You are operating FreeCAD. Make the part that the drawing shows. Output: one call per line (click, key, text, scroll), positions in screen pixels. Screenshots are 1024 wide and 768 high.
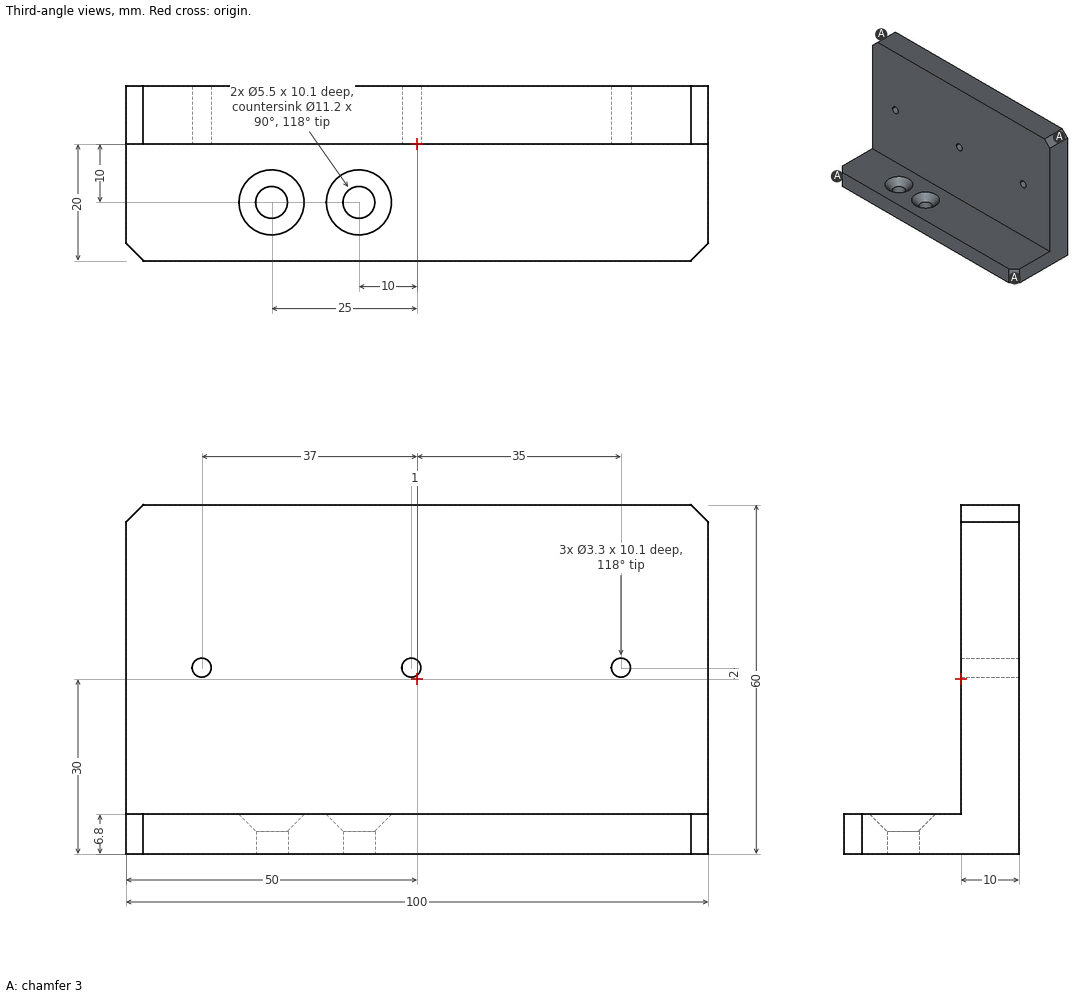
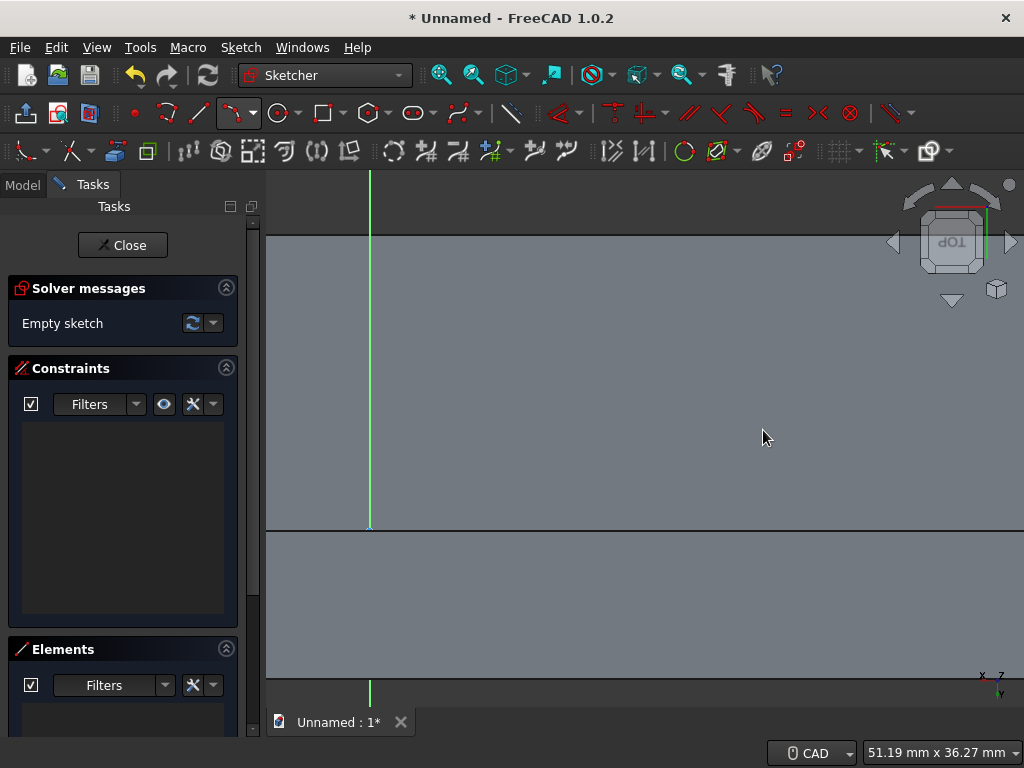
key(g)
key(c)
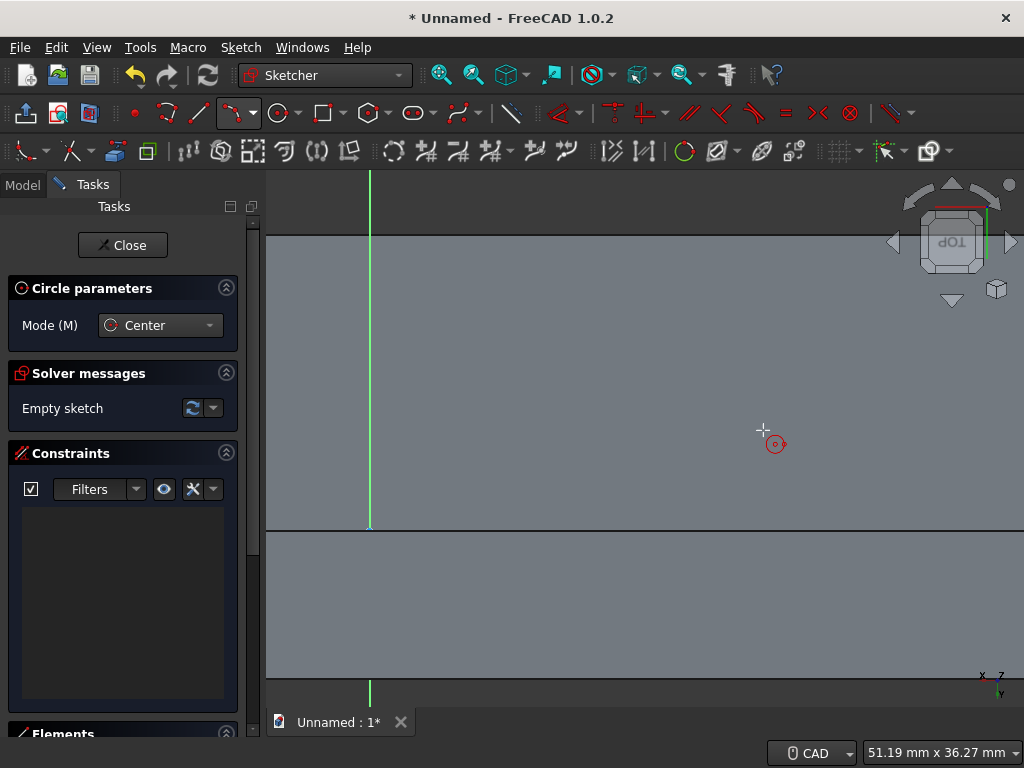
click(518, 383)
click(547, 354)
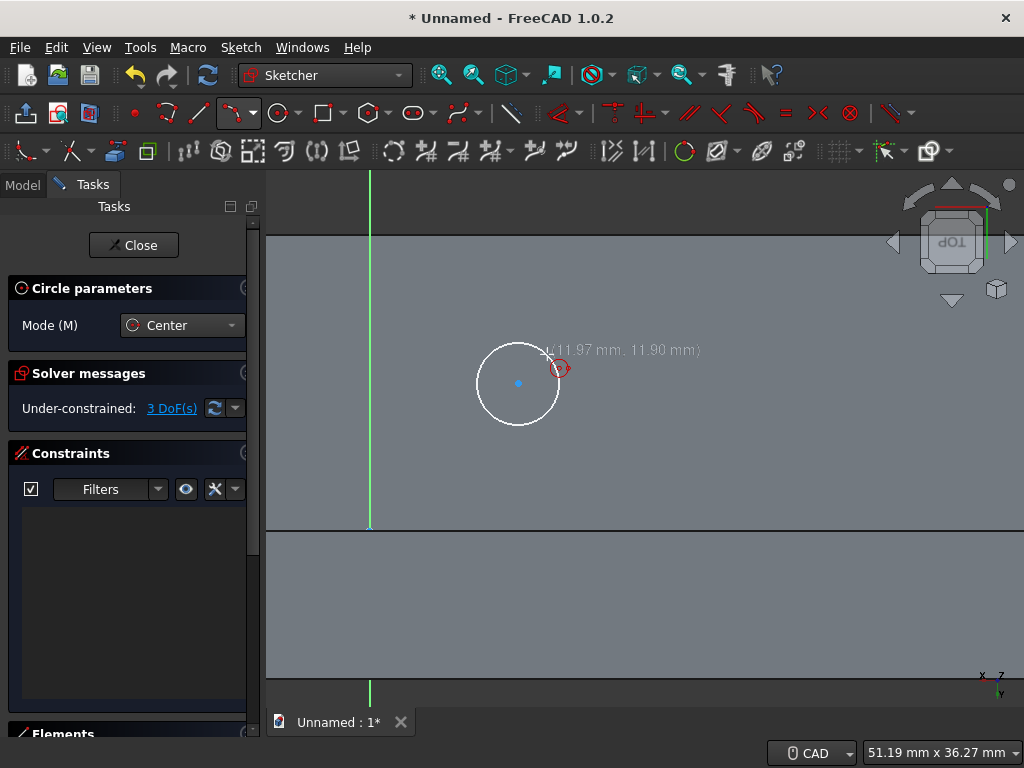
click(740, 383)
click(769, 354)
key(Escape)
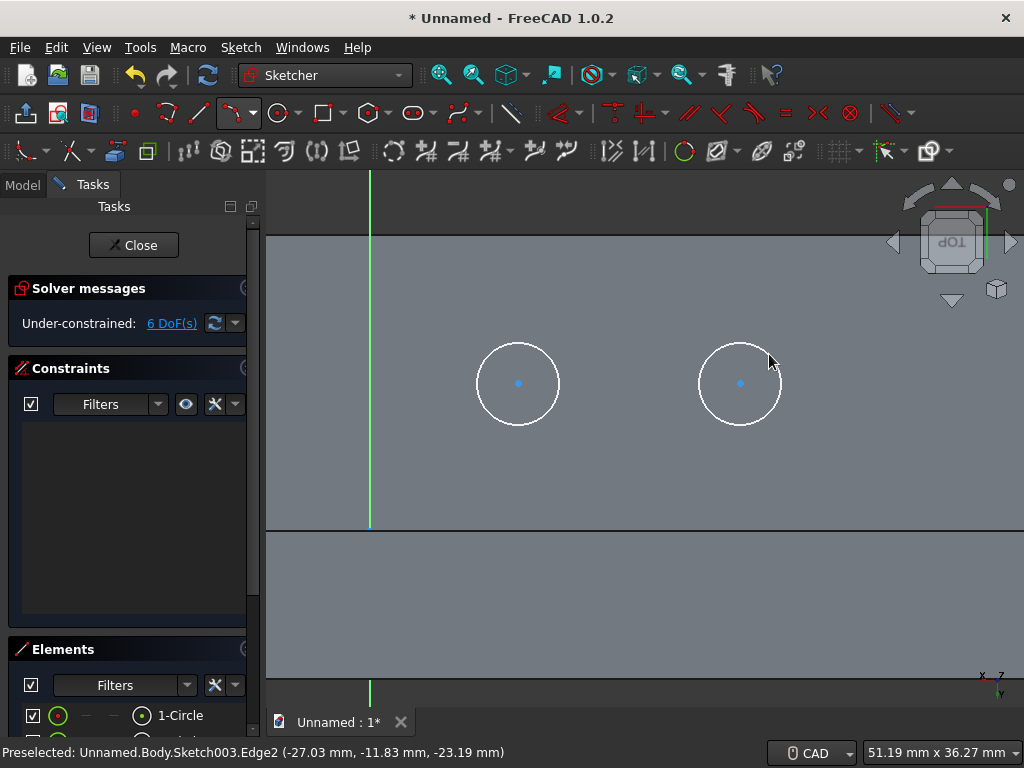
click(547, 355)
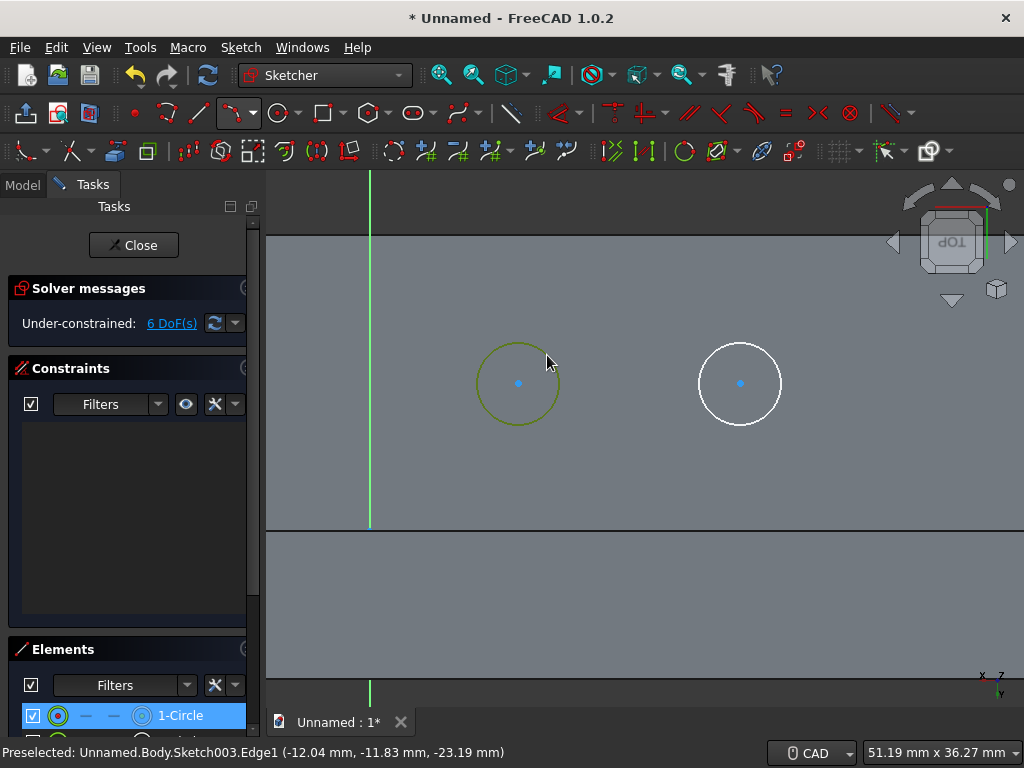
click(769, 355)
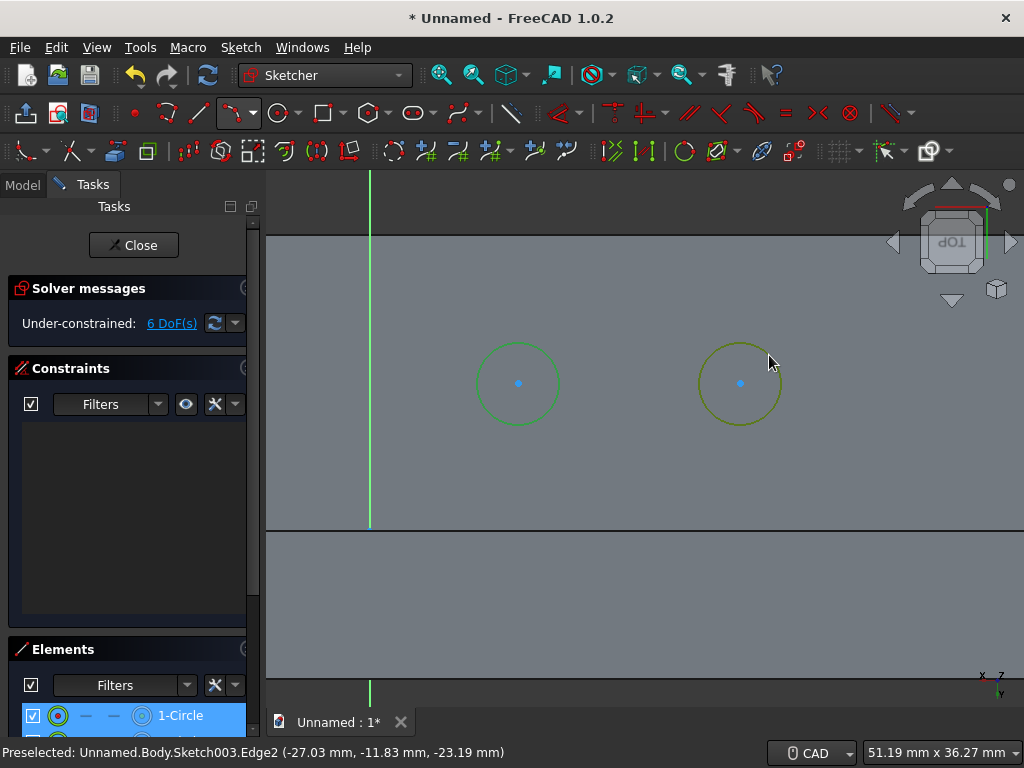
click(786, 114)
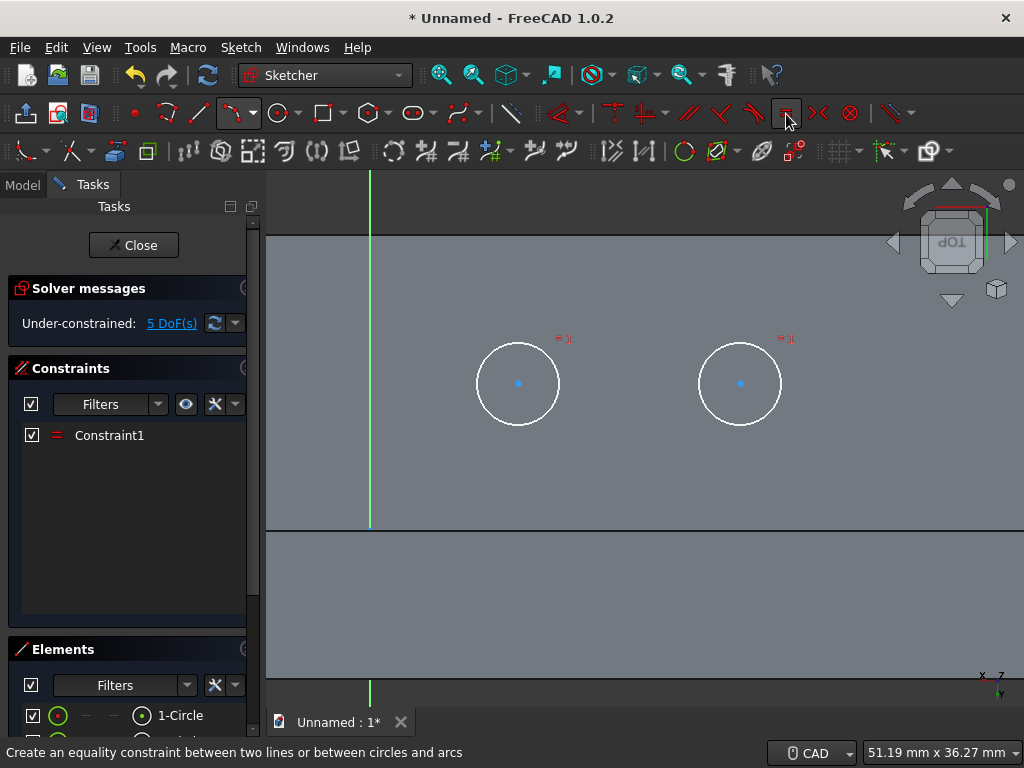
click(518, 384)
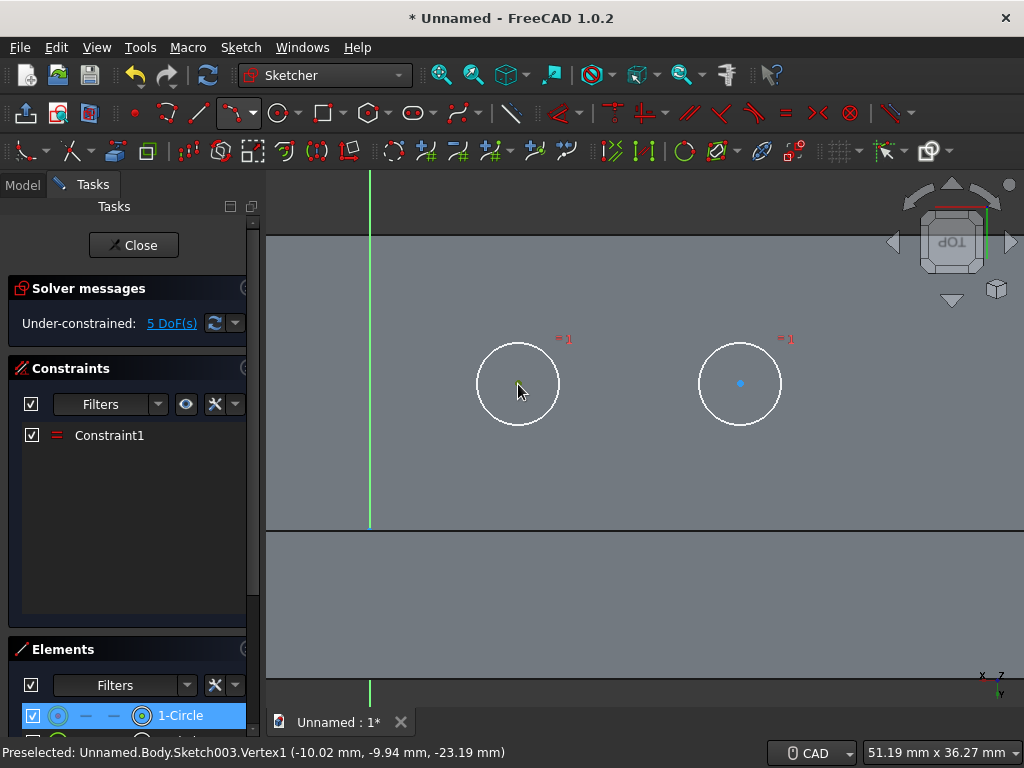
click(740, 384)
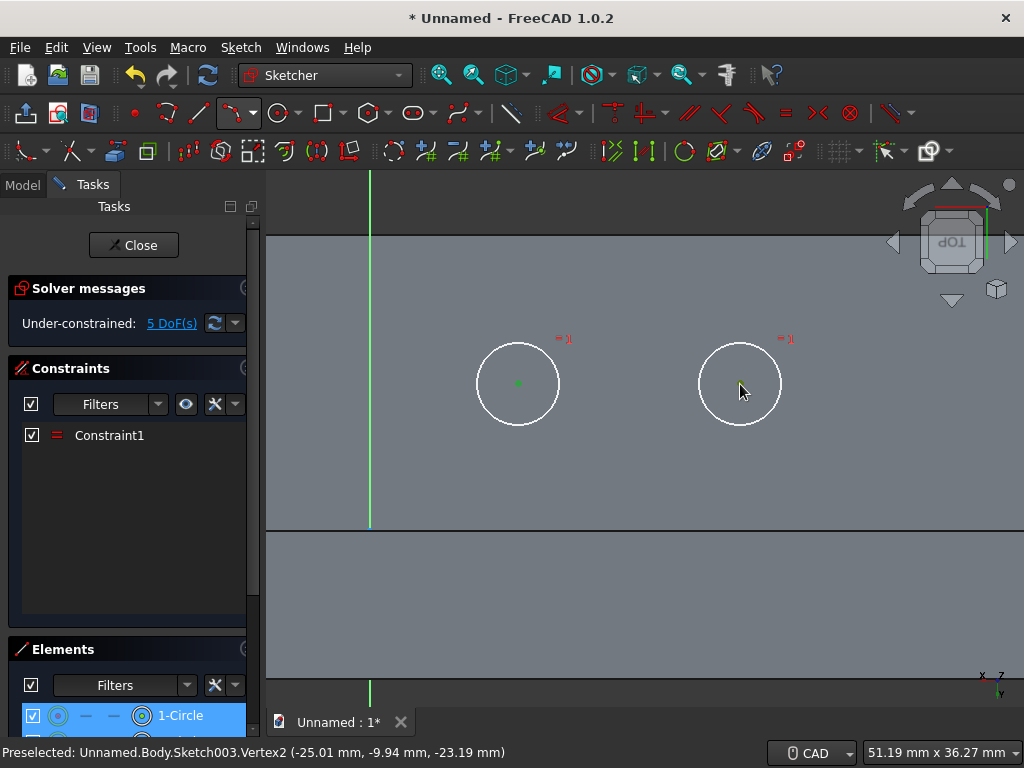
key(h)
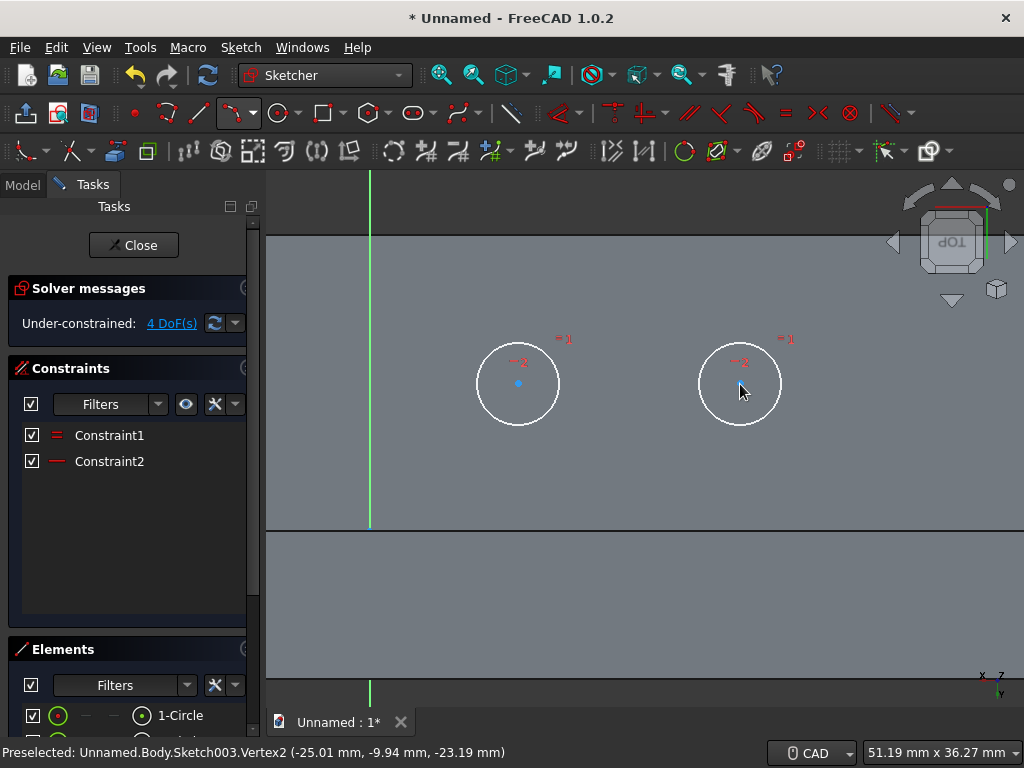
key(d)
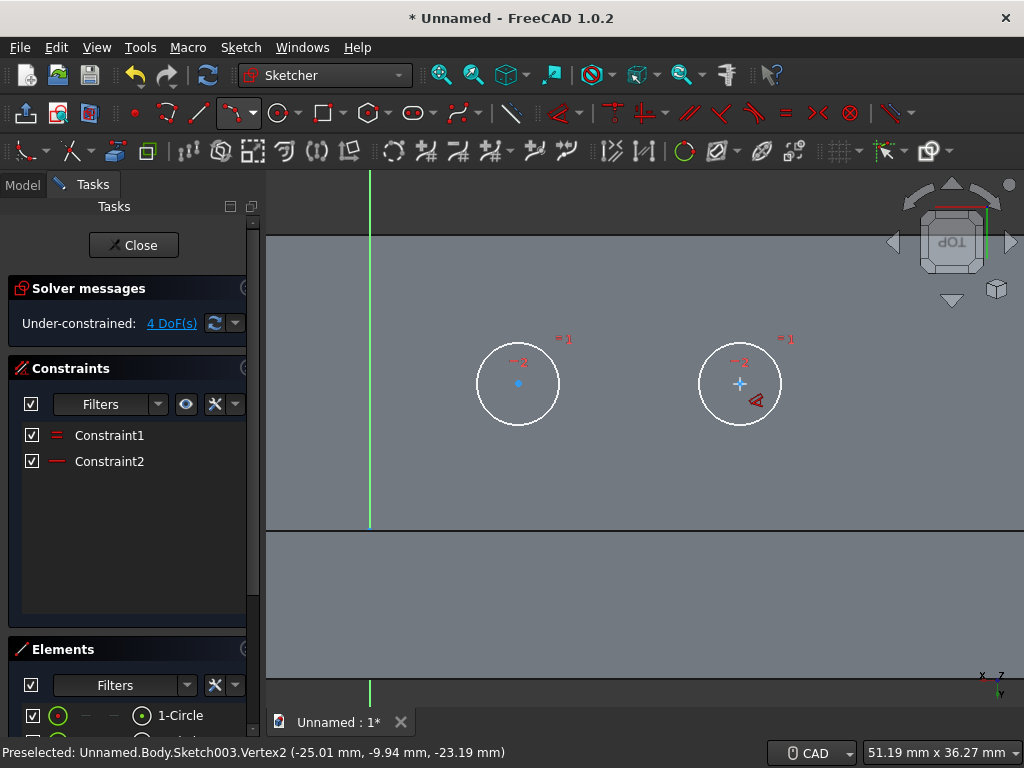
click(547, 355)
click(570, 332)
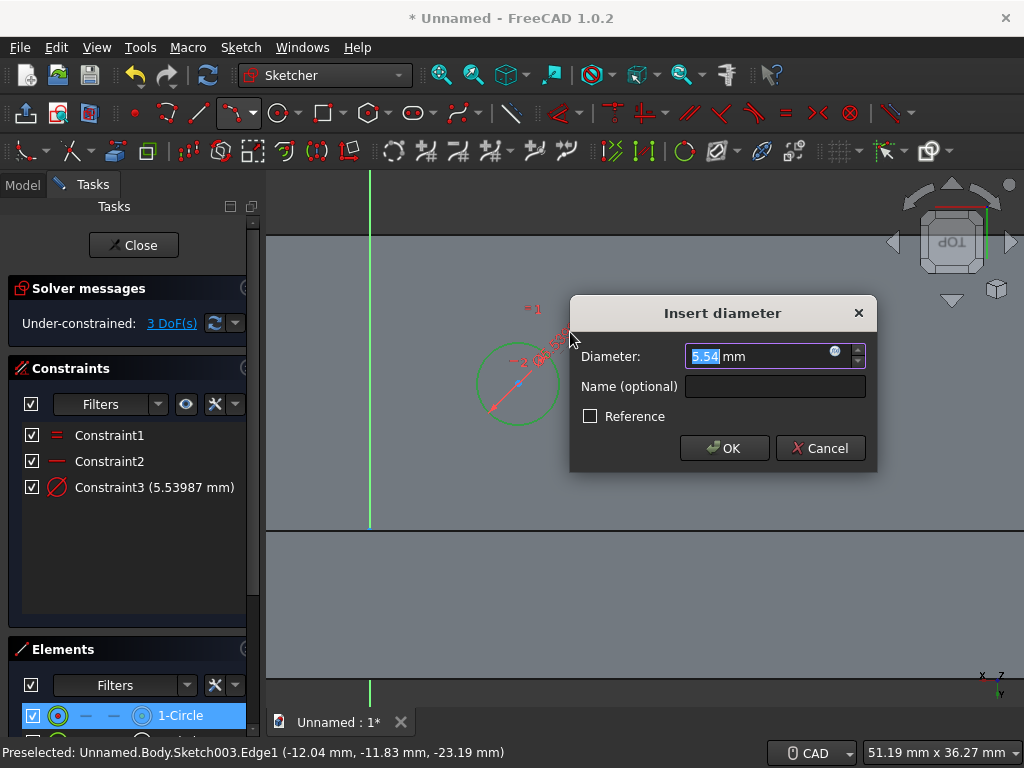
text(5.5)
key(Return)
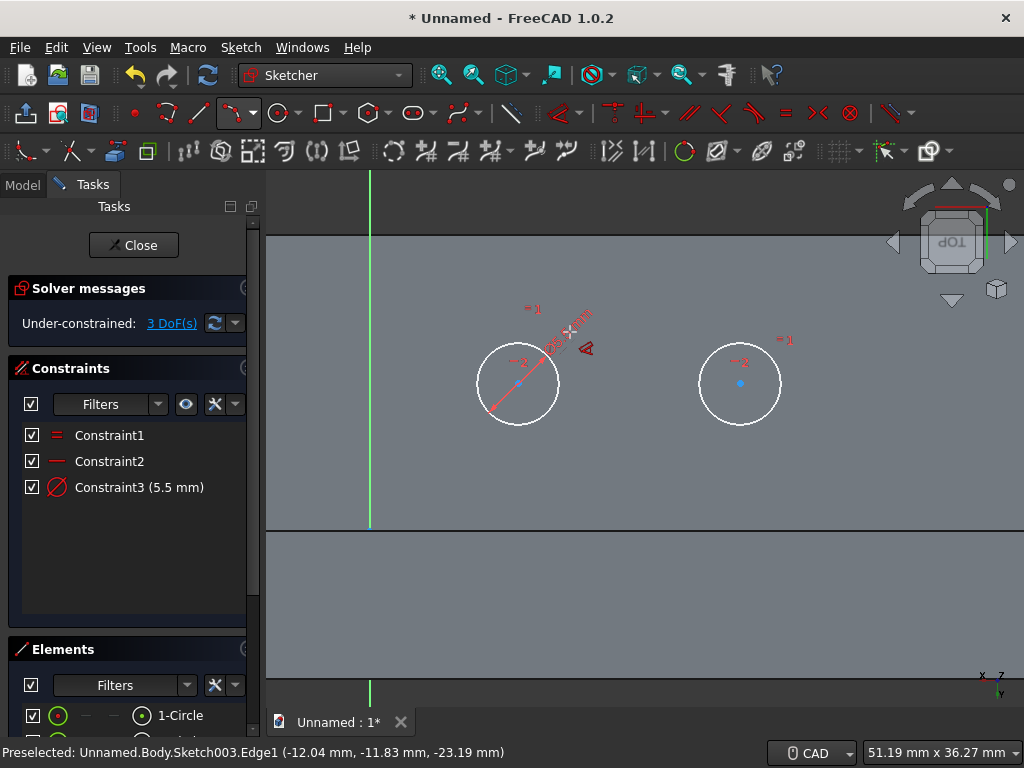
click(518, 384)
click(444, 565)